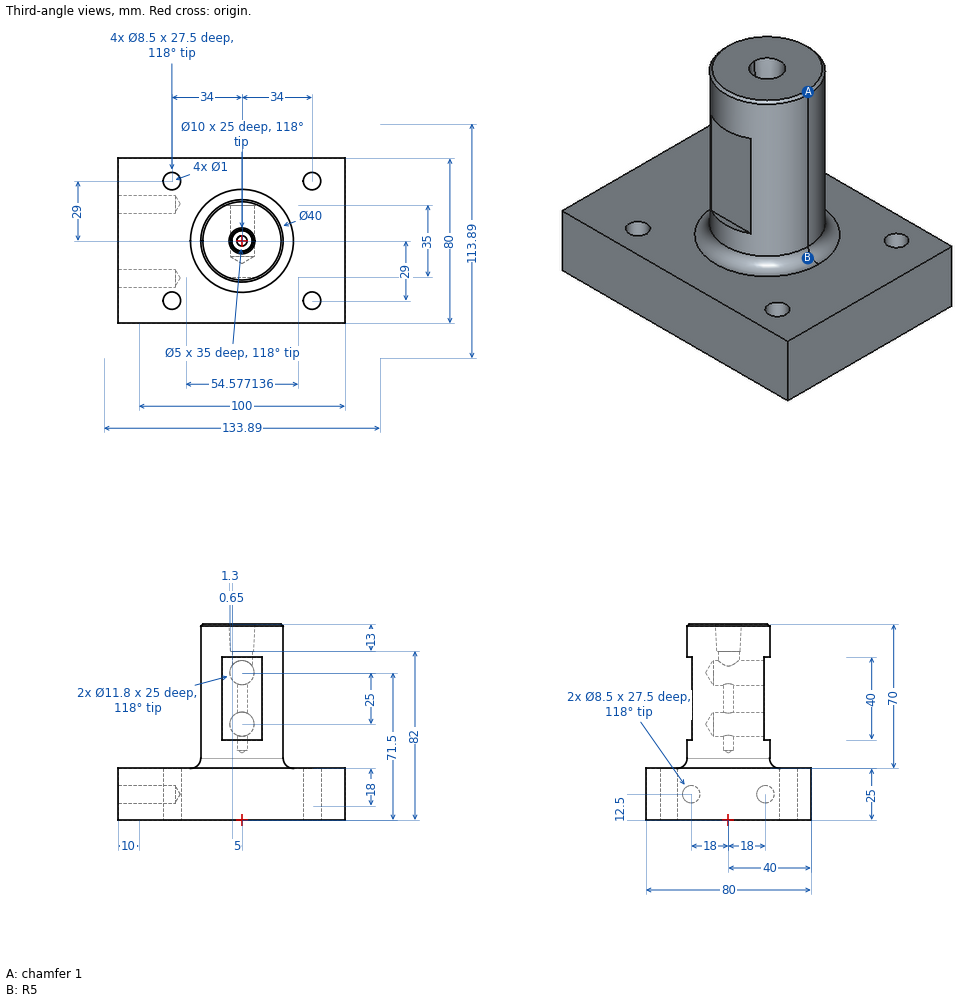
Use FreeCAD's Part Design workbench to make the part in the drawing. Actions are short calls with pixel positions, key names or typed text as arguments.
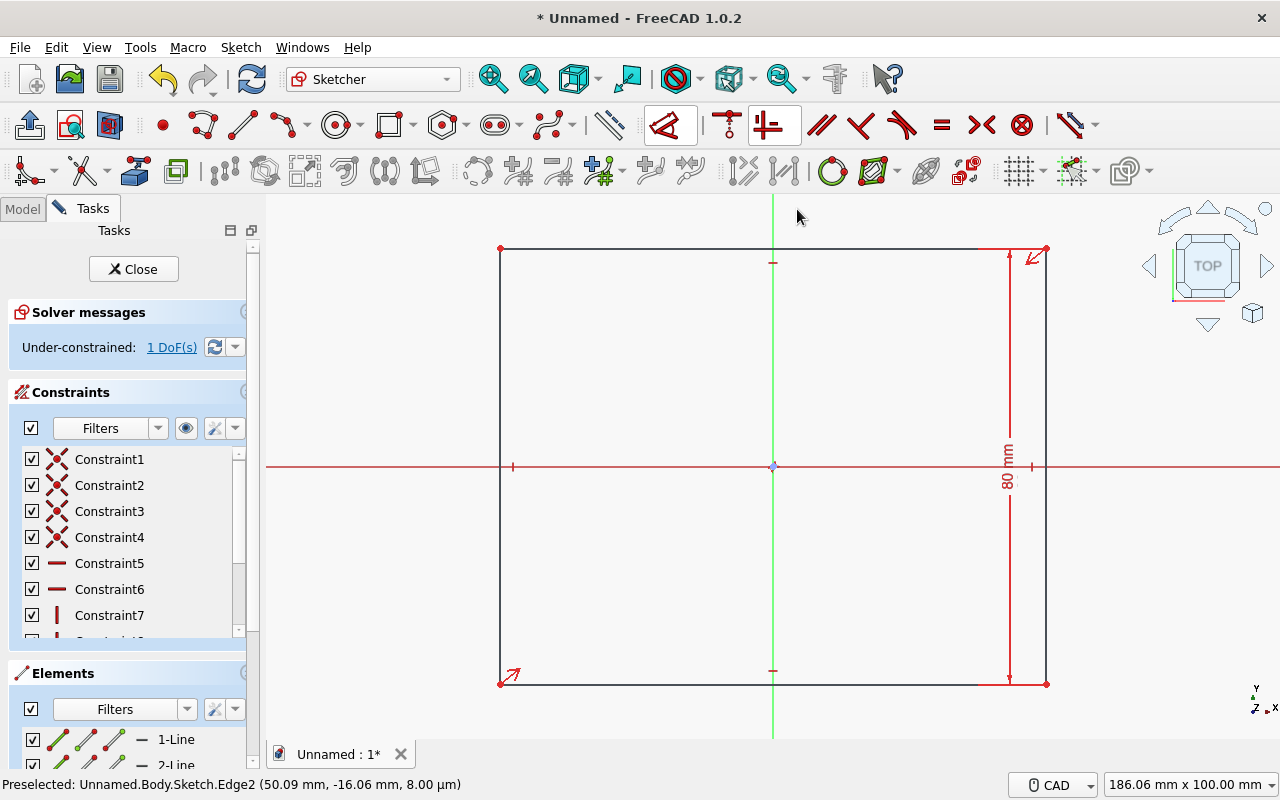
click(664, 684)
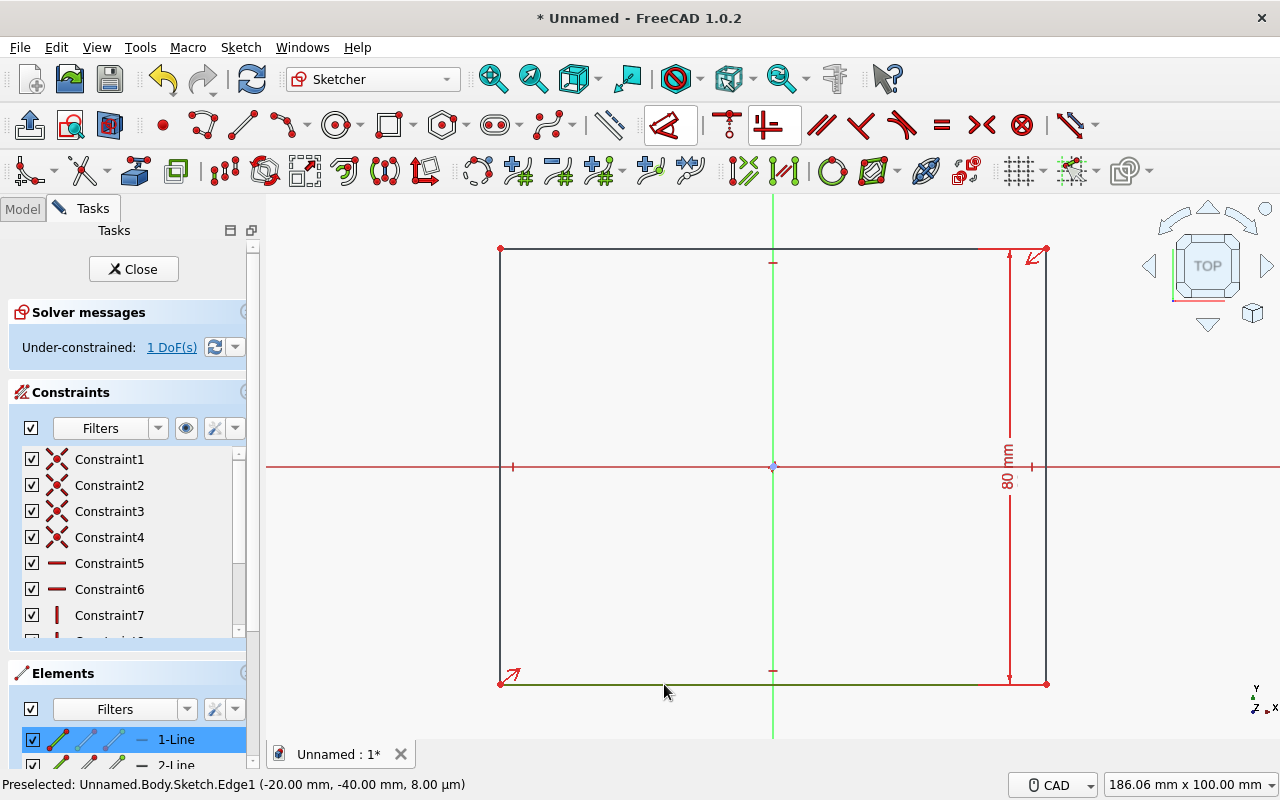
key(l)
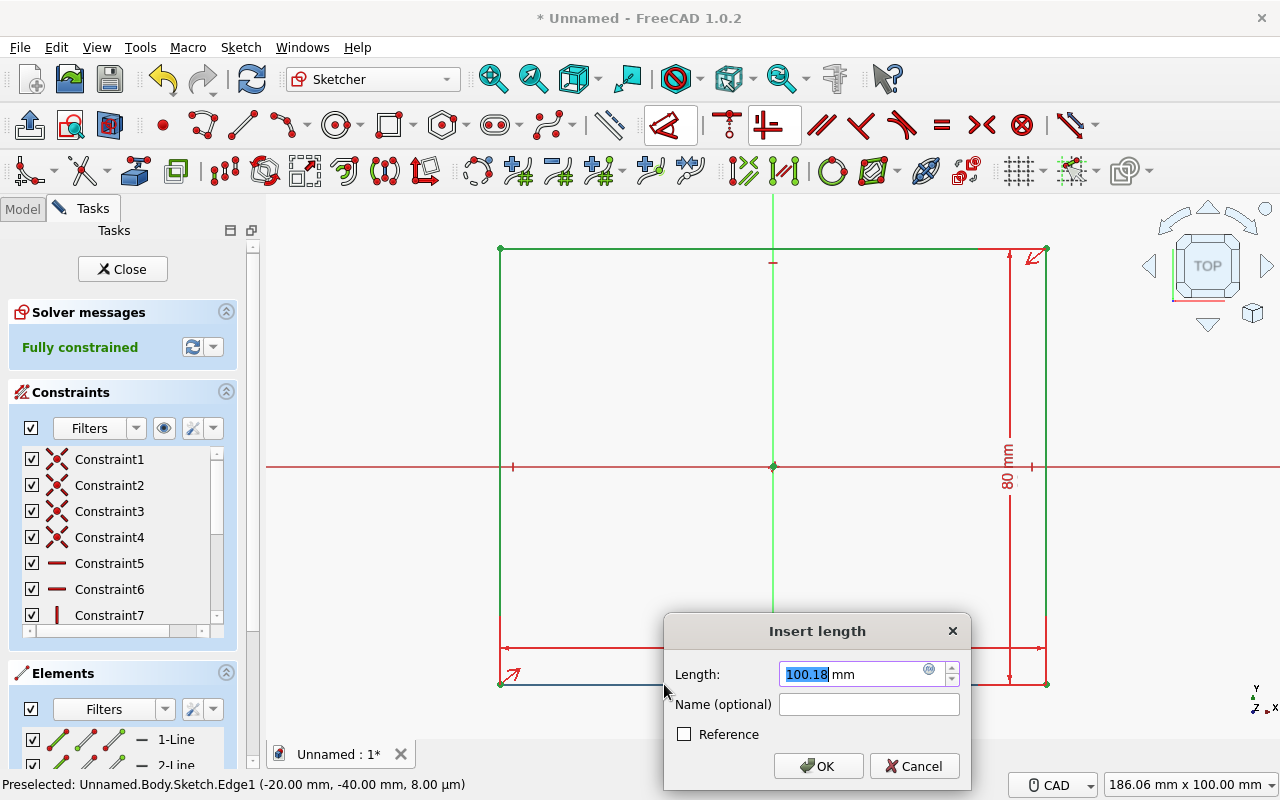
text(100)
key(Return)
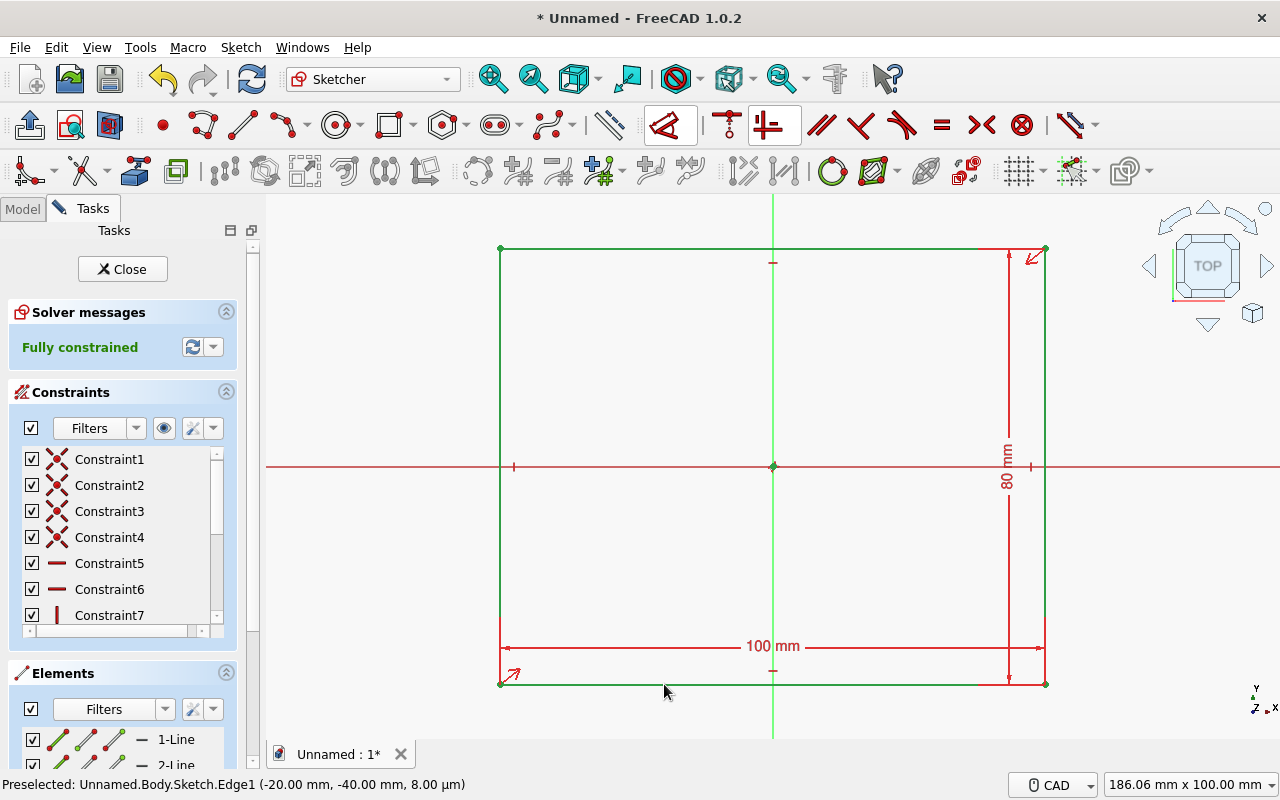
click(123, 269)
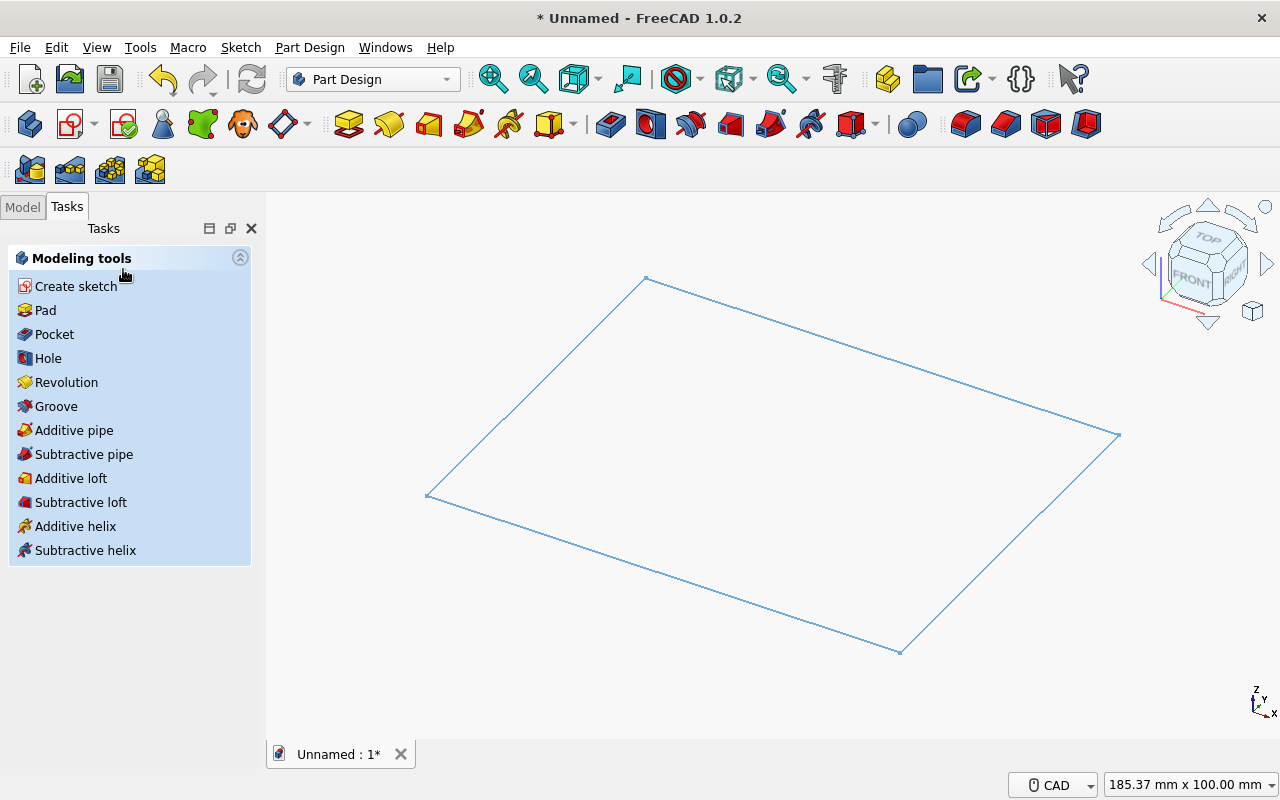
click(350, 124)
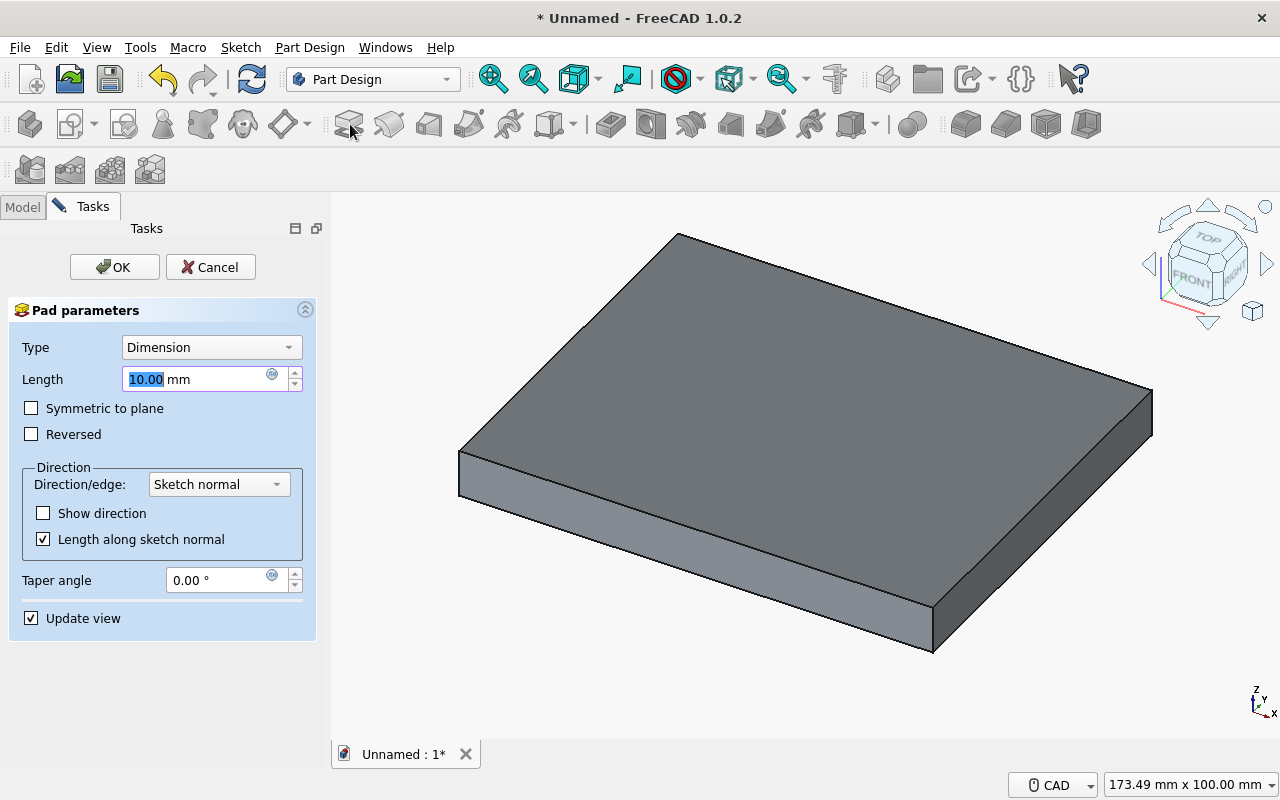
text(25)
key(Tab)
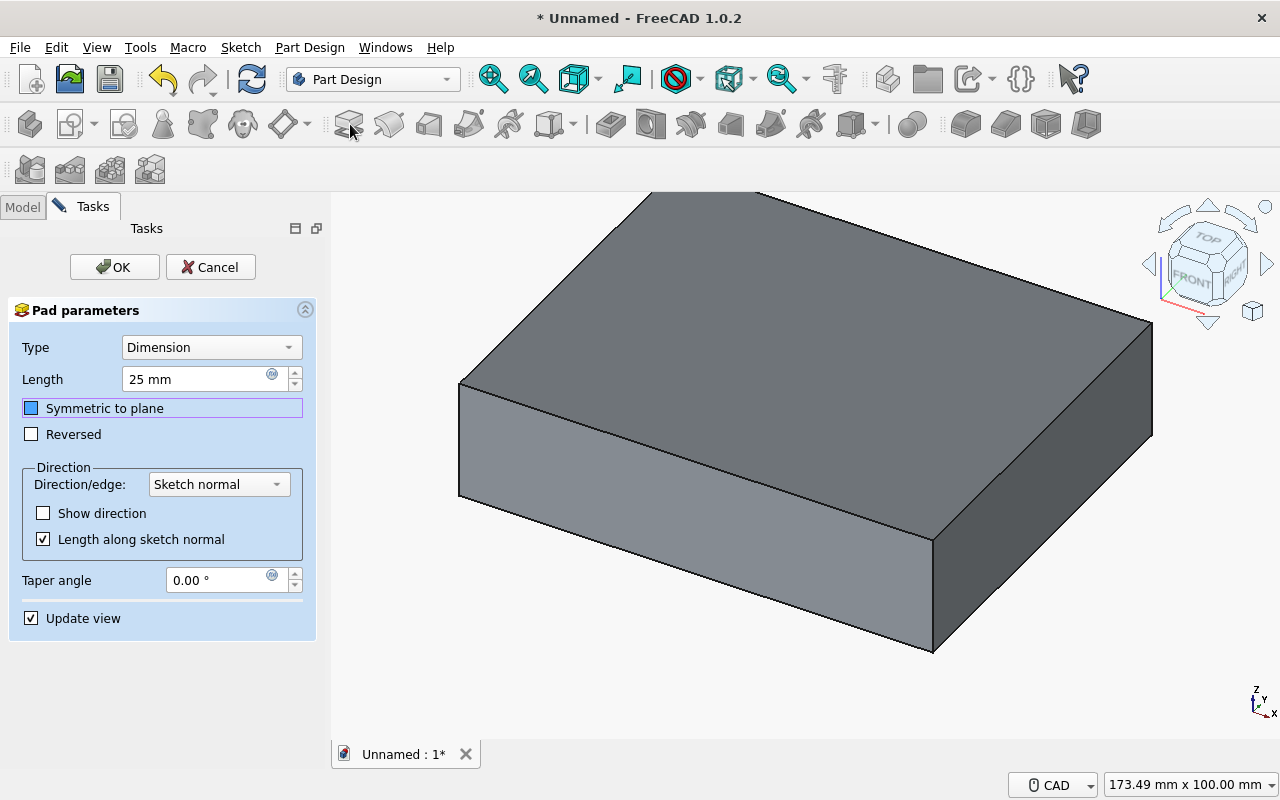
click(115, 267)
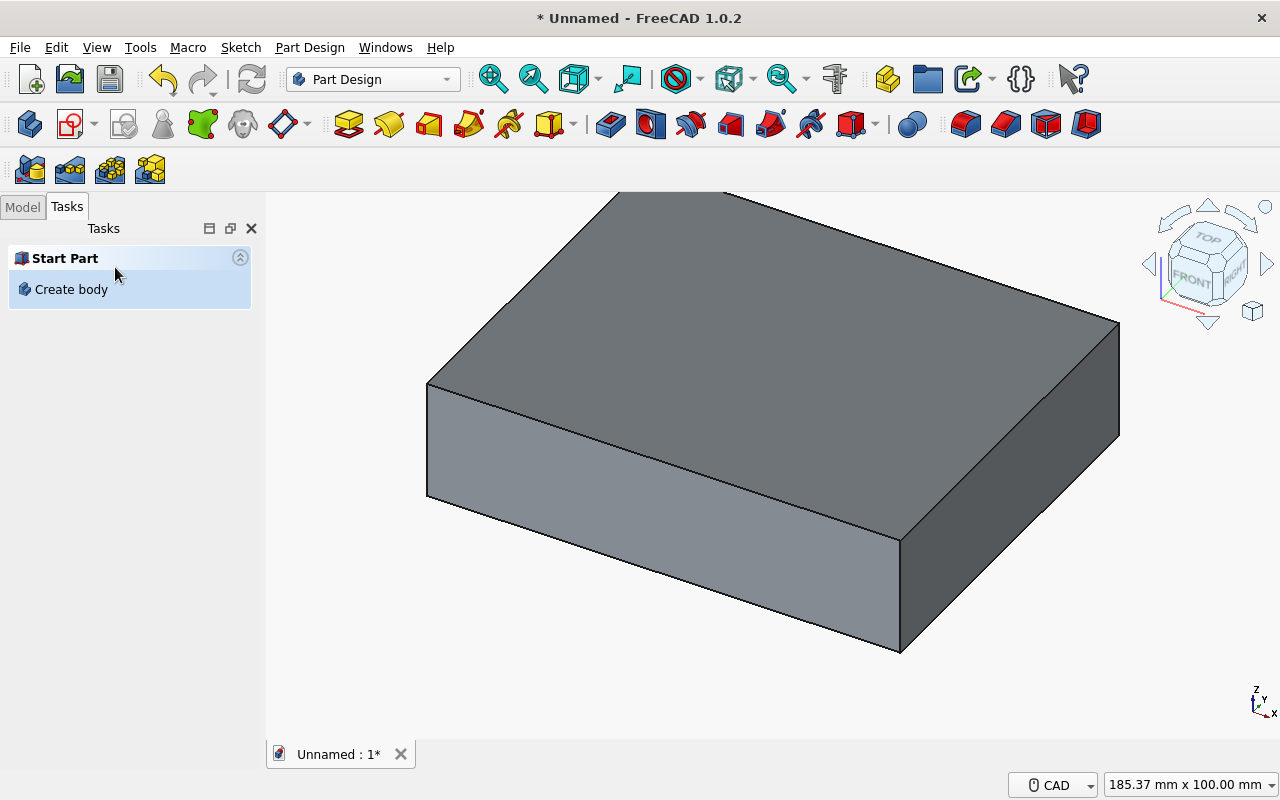
click(494, 80)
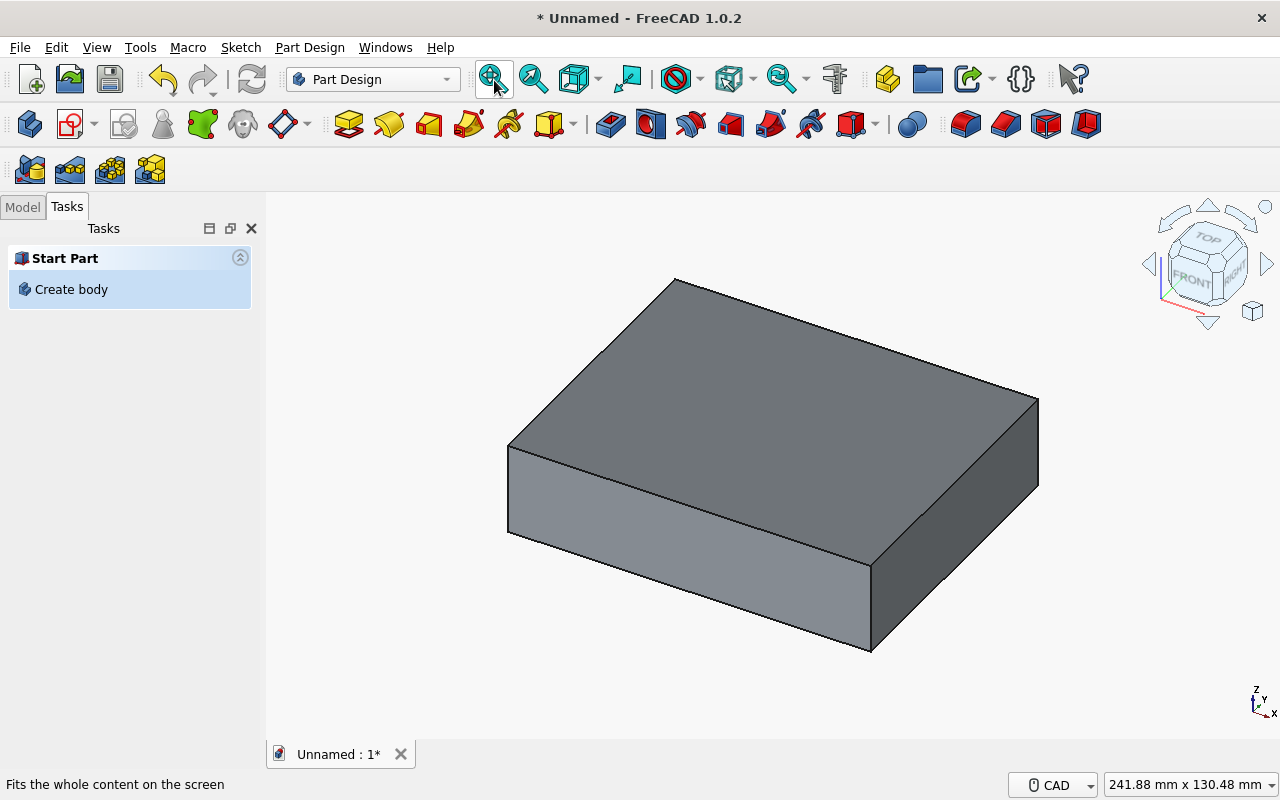
click(773, 422)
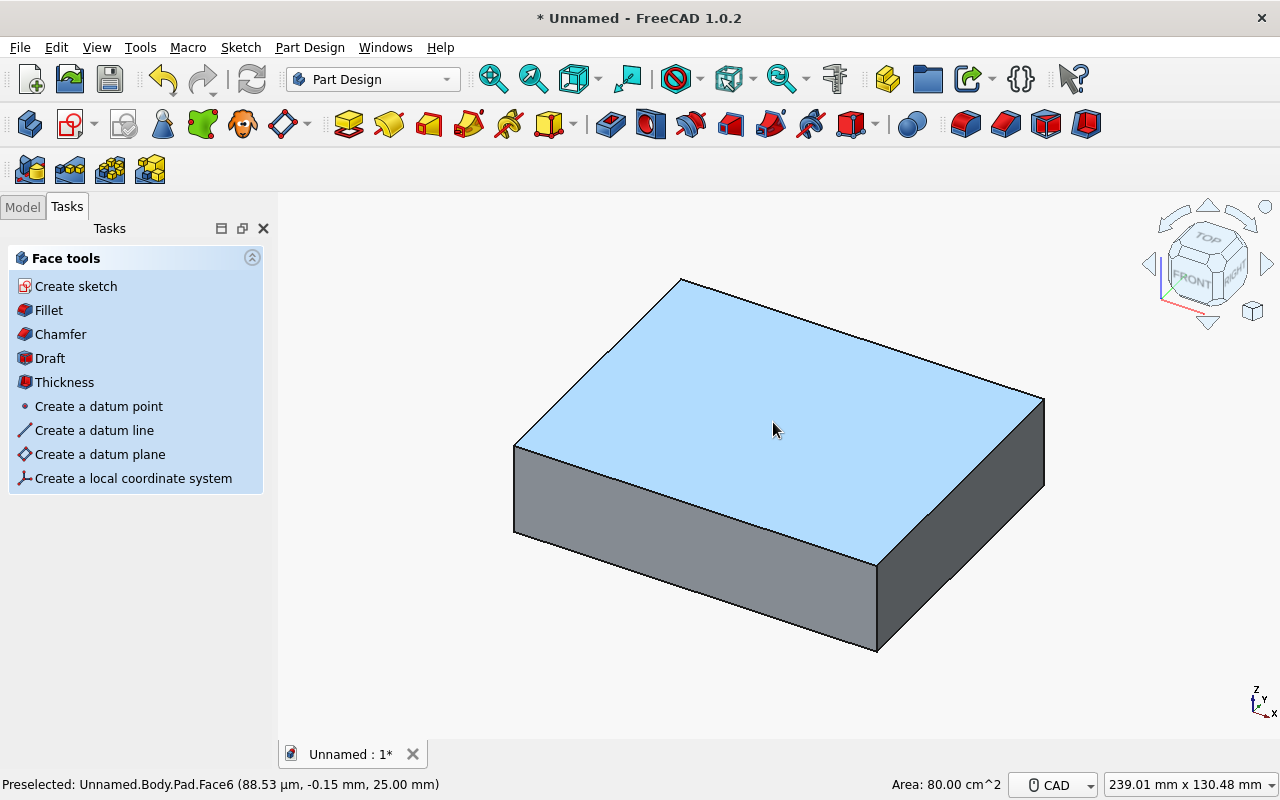
click(70, 124)